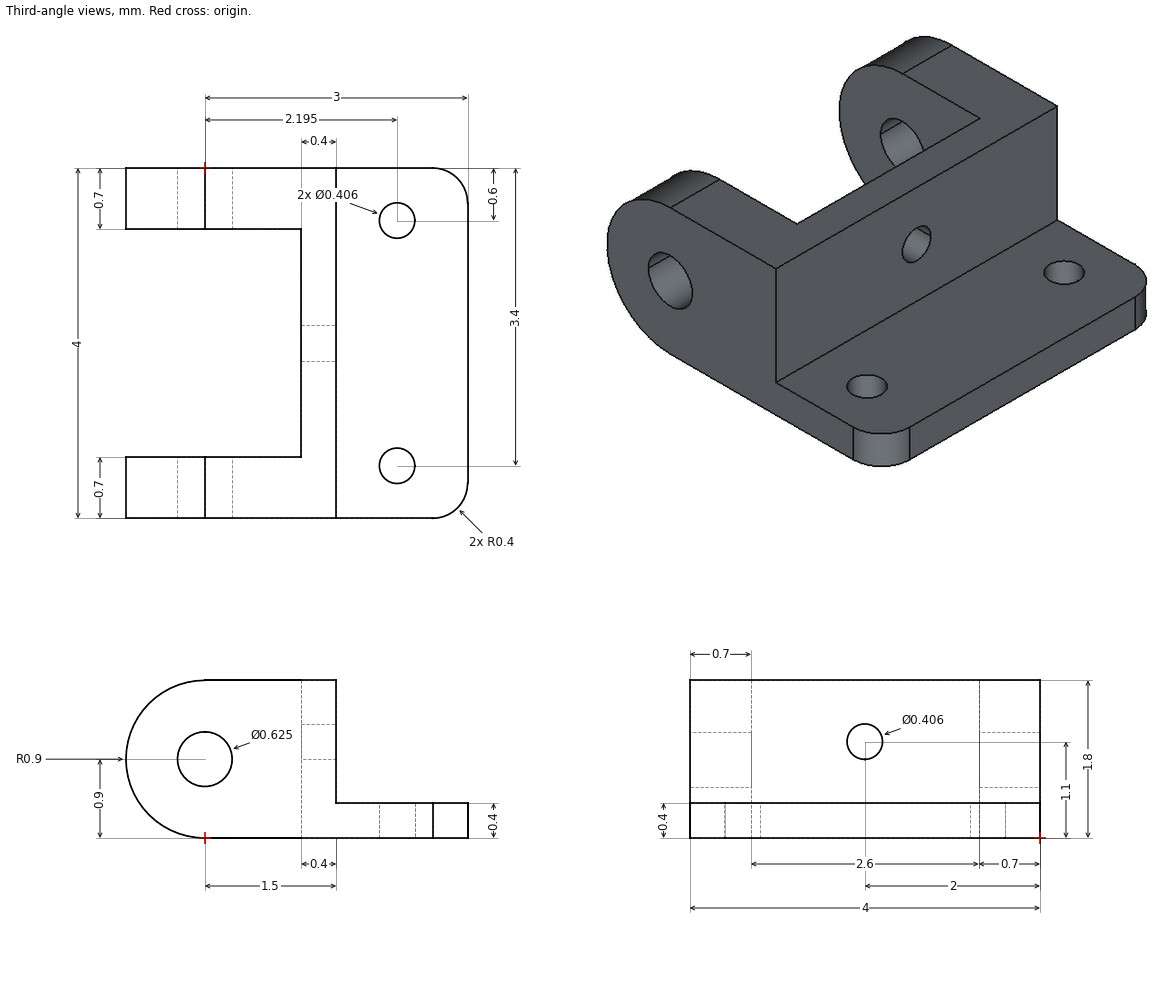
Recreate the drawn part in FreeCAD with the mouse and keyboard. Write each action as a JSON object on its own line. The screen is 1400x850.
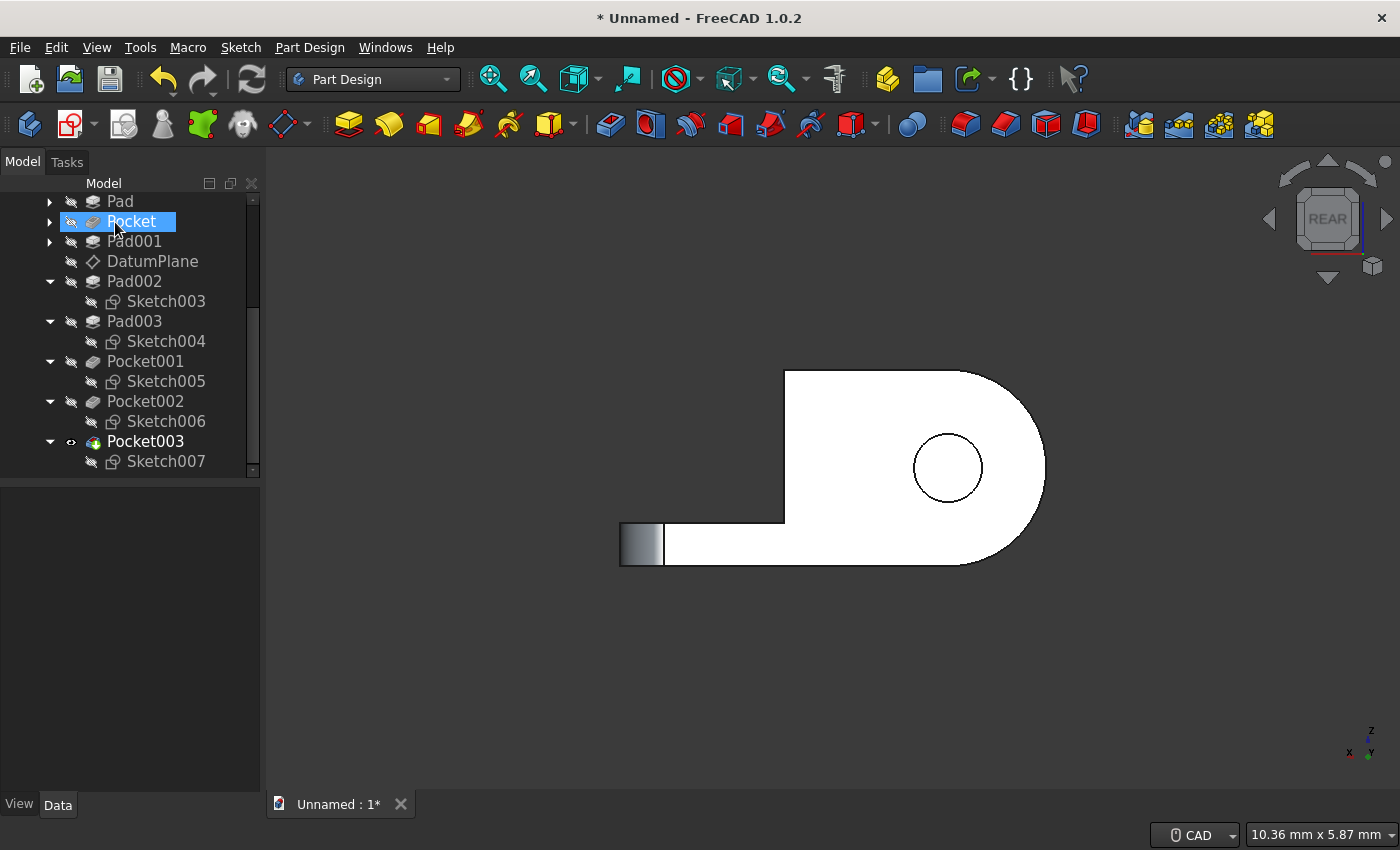
{"action": "left_click", "coordinate": [937, 467]}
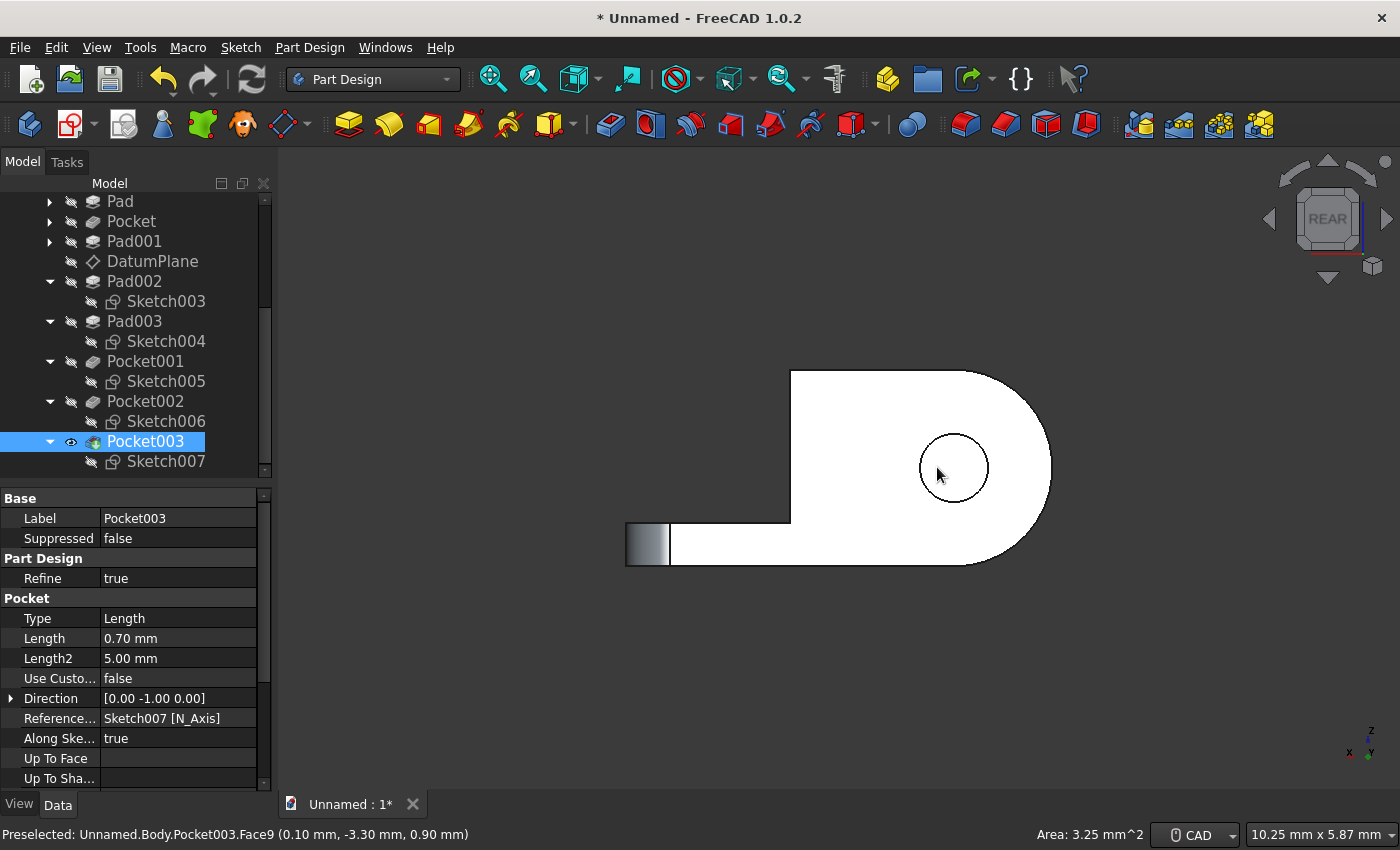
{"action": "left_click", "coordinate": [70, 124]}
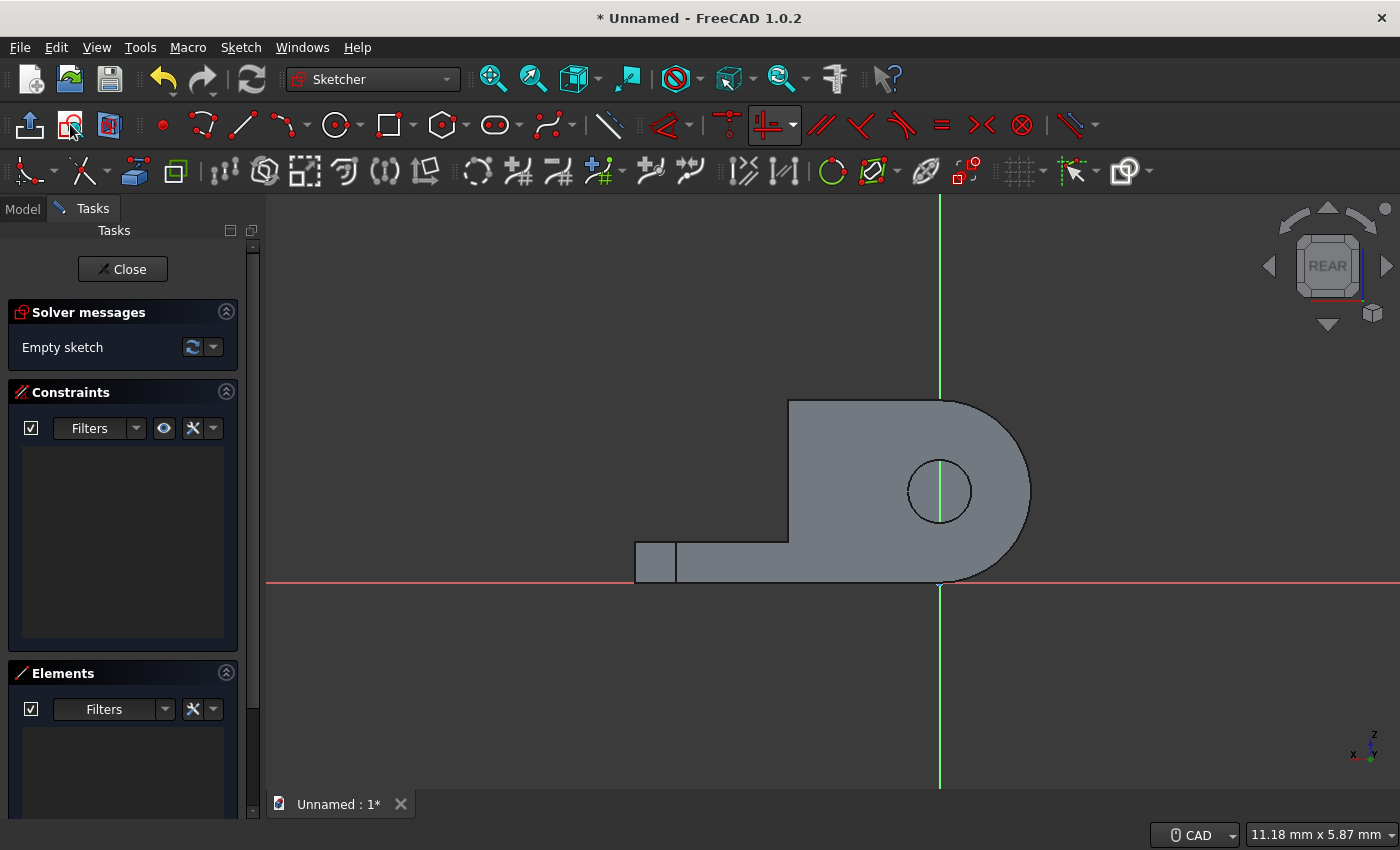
{"action": "key", "text": "q s"}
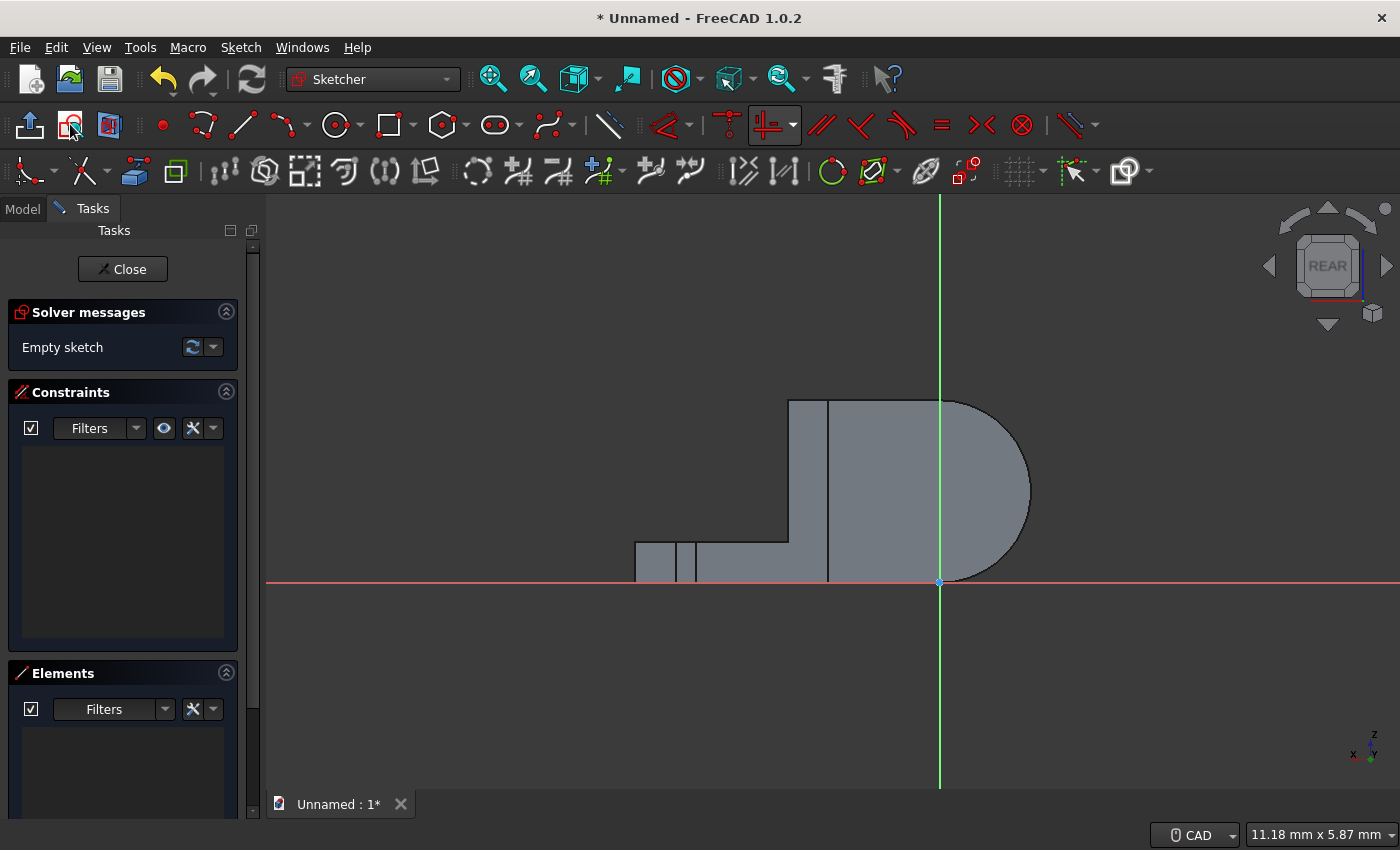
{"action": "scroll", "coordinate": [1015, 534], "scroll_direction": "up", "scroll_amount": 6}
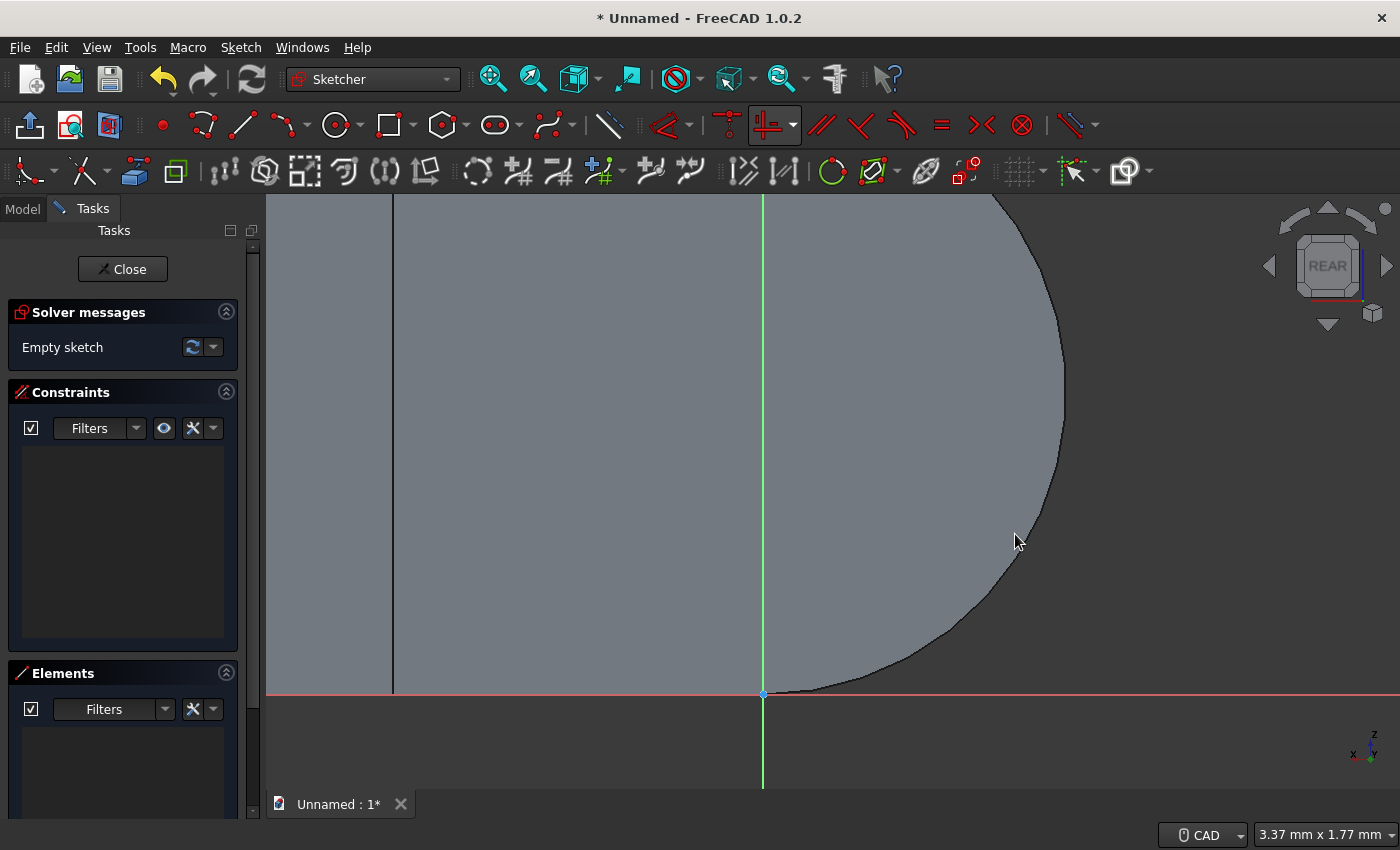
{"action": "key", "text": "g c"}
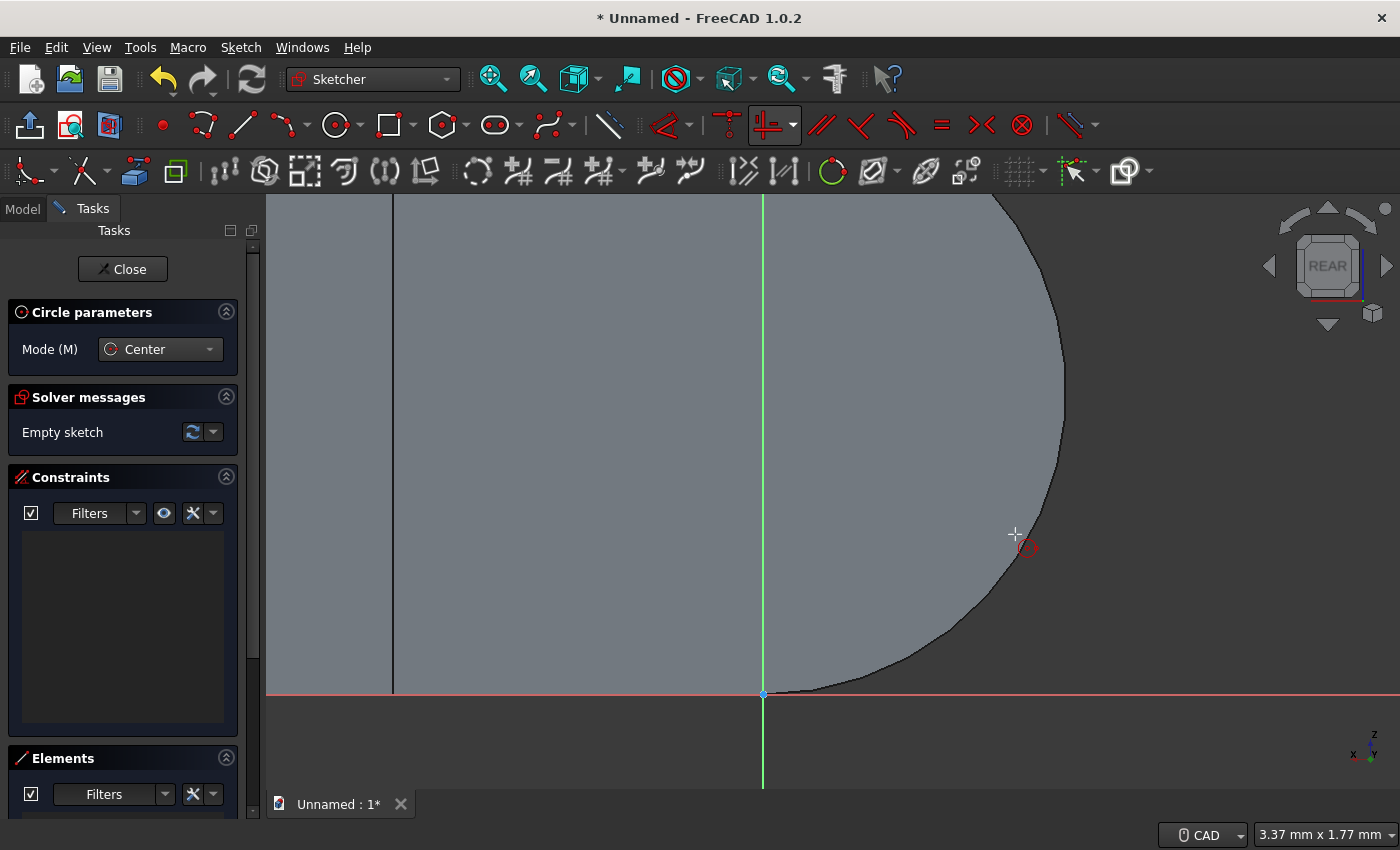
{"action": "left_click", "coordinate": [763, 392]}
{"action": "mouse_move", "coordinate": [838, 317]}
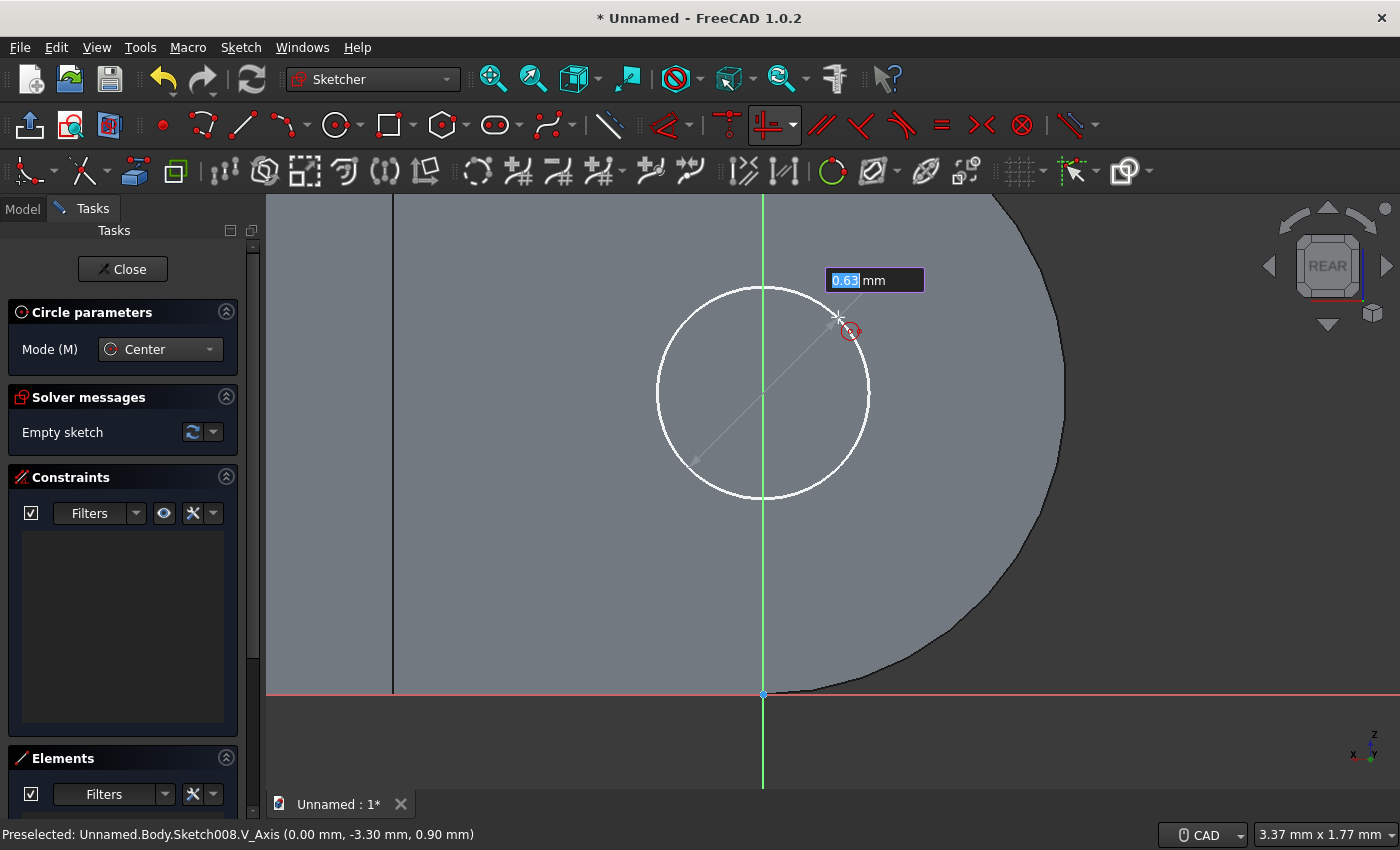
{"action": "type", "text": "0.625"}
{"action": "key", "text": "Return"}
{"action": "key", "text": "Escape"}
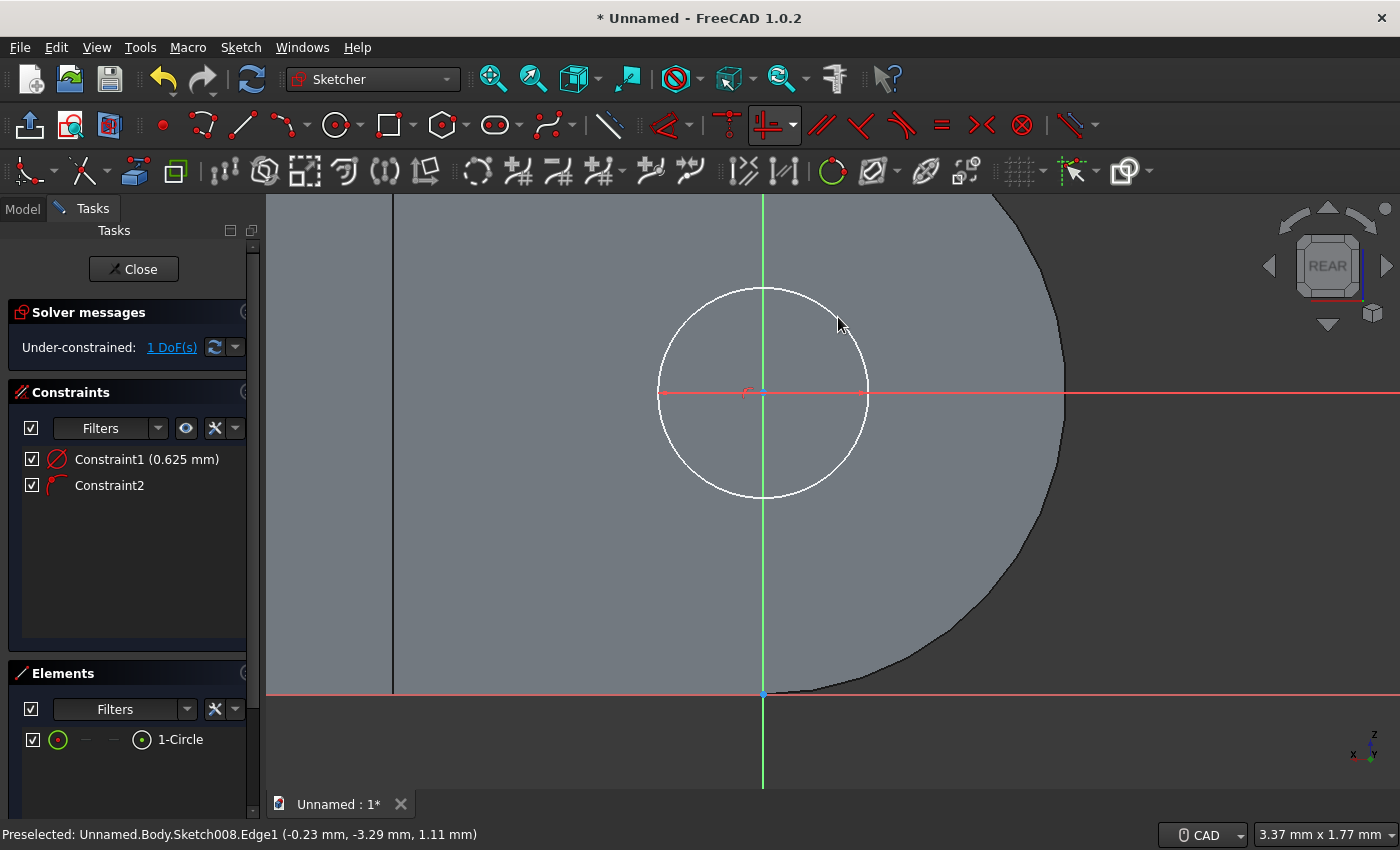
{"action": "left_click", "coordinate": [664, 126]}